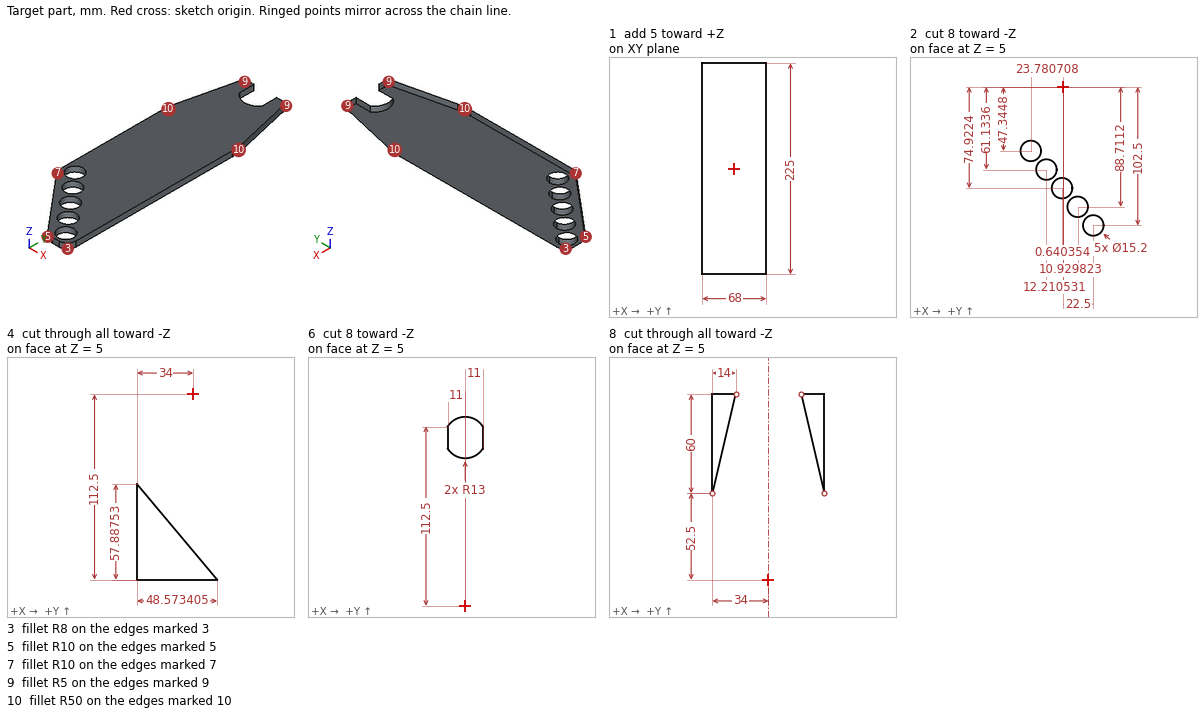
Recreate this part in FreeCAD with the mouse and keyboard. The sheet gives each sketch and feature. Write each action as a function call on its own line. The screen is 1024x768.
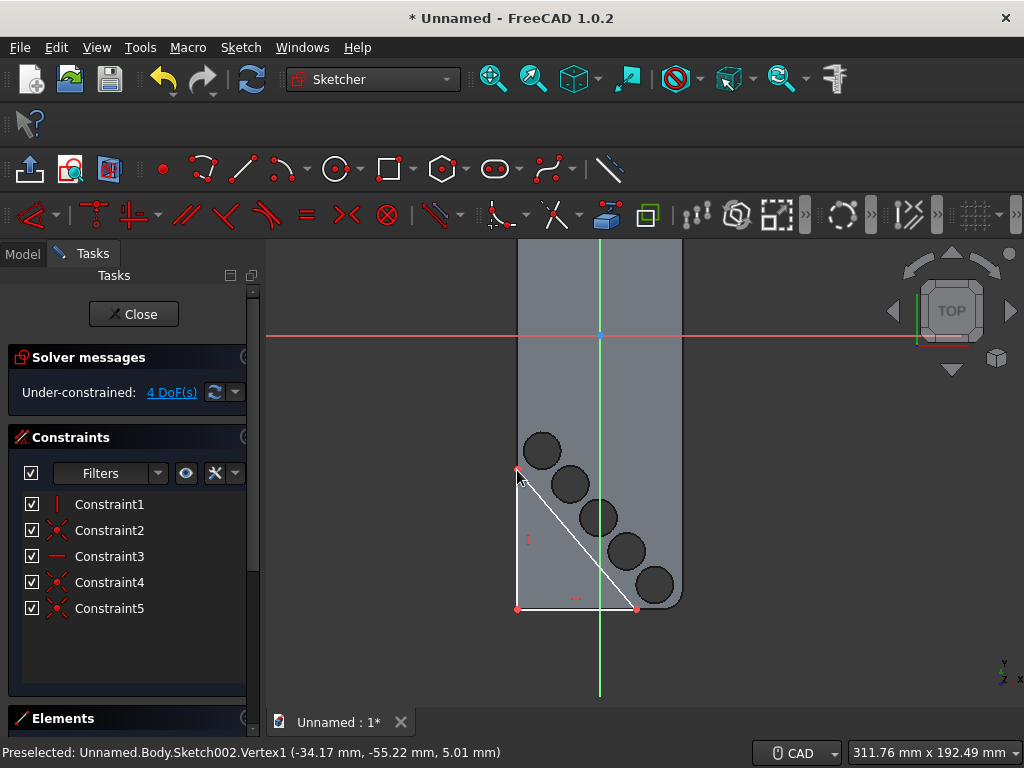
click(32, 216)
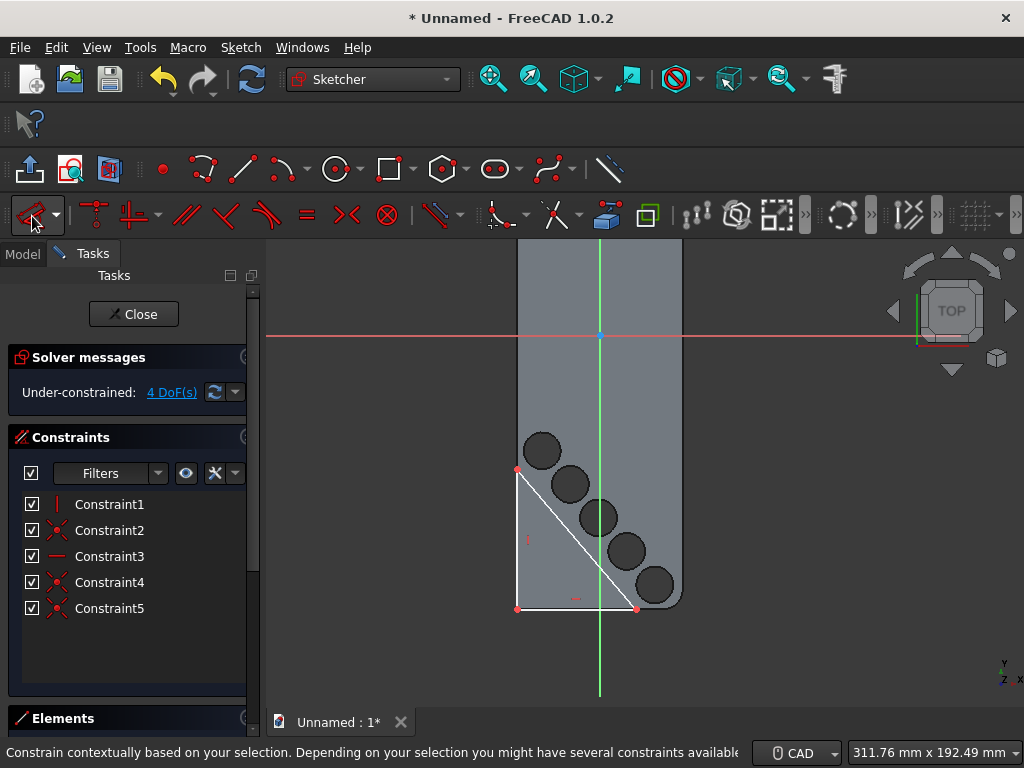
click(517, 470)
click(559, 302)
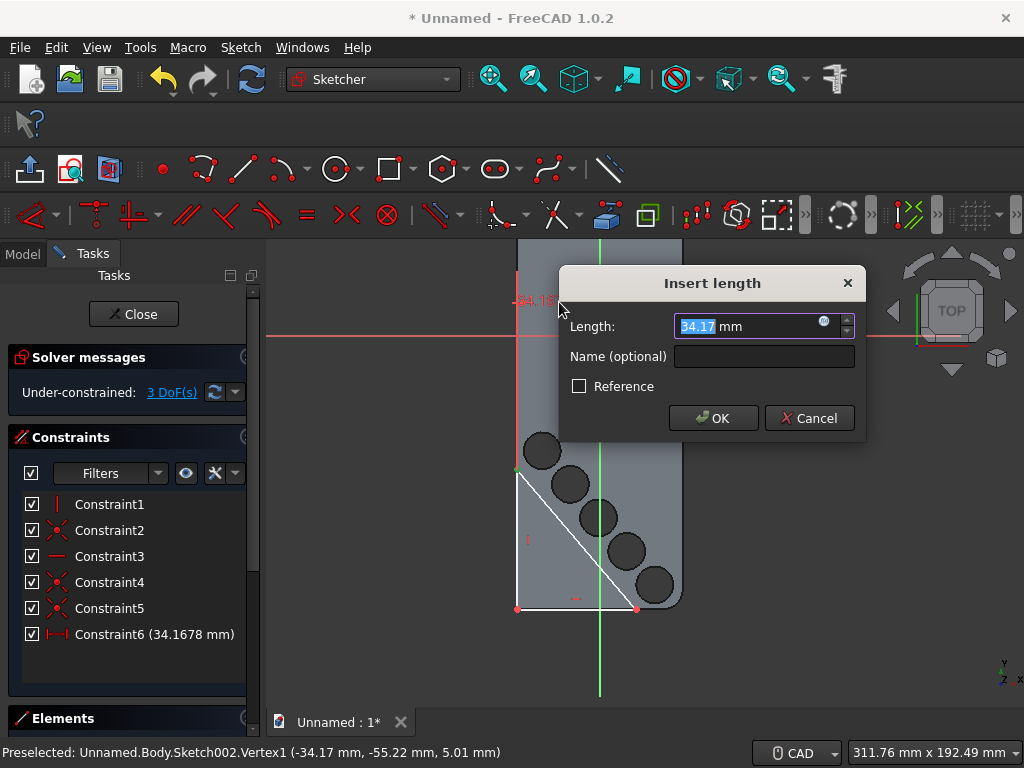
text(34)
key(Return)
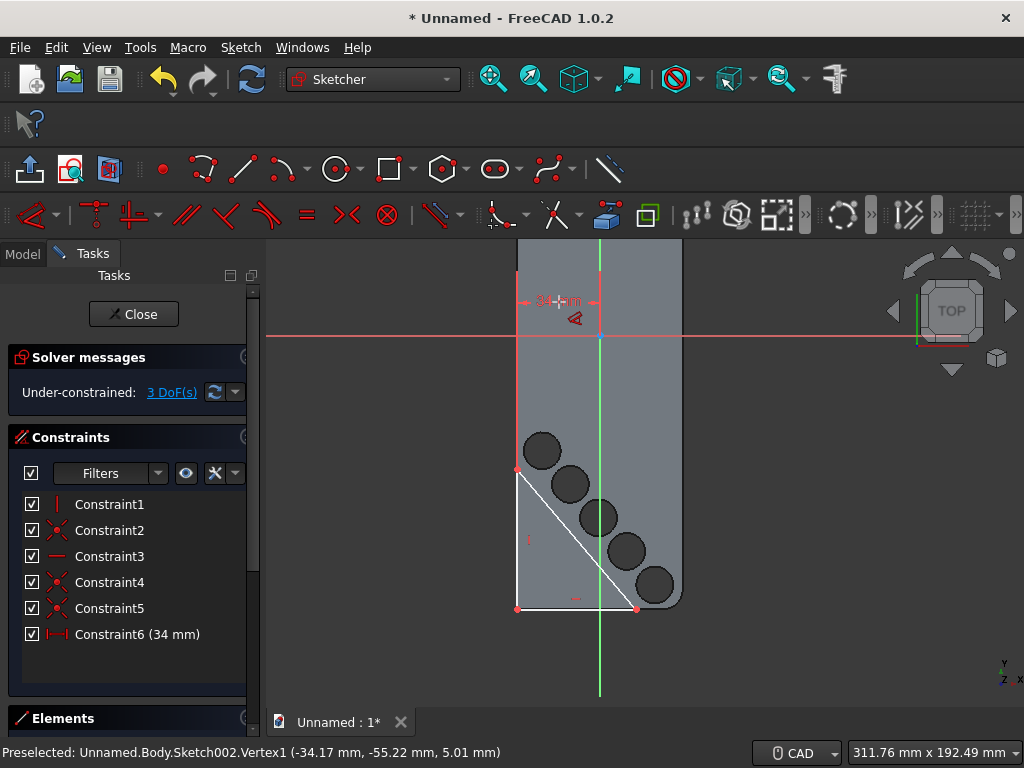
click(517, 610)
click(483, 473)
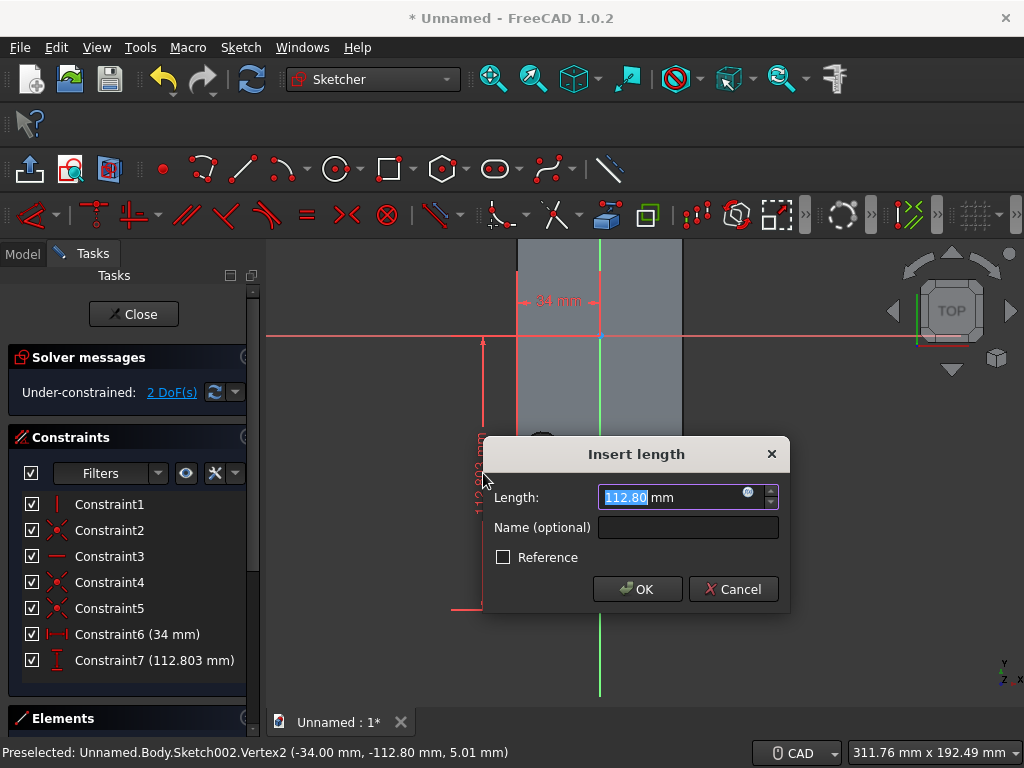
text(112.5)
key(Return)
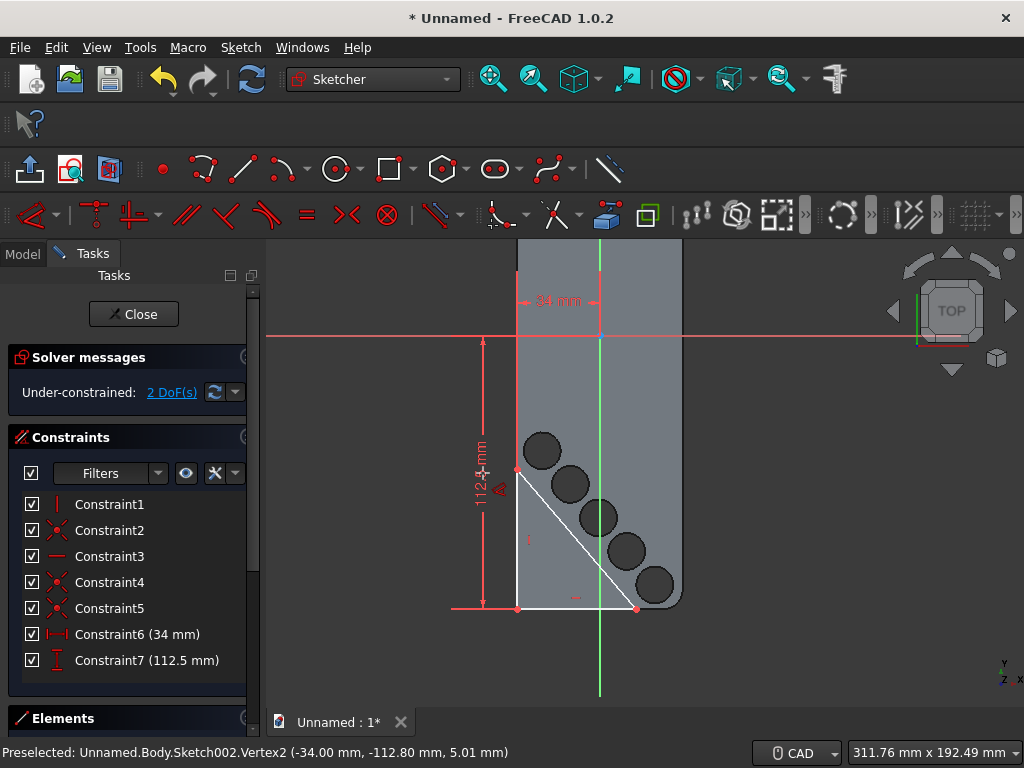
click(517, 512)
click(483, 540)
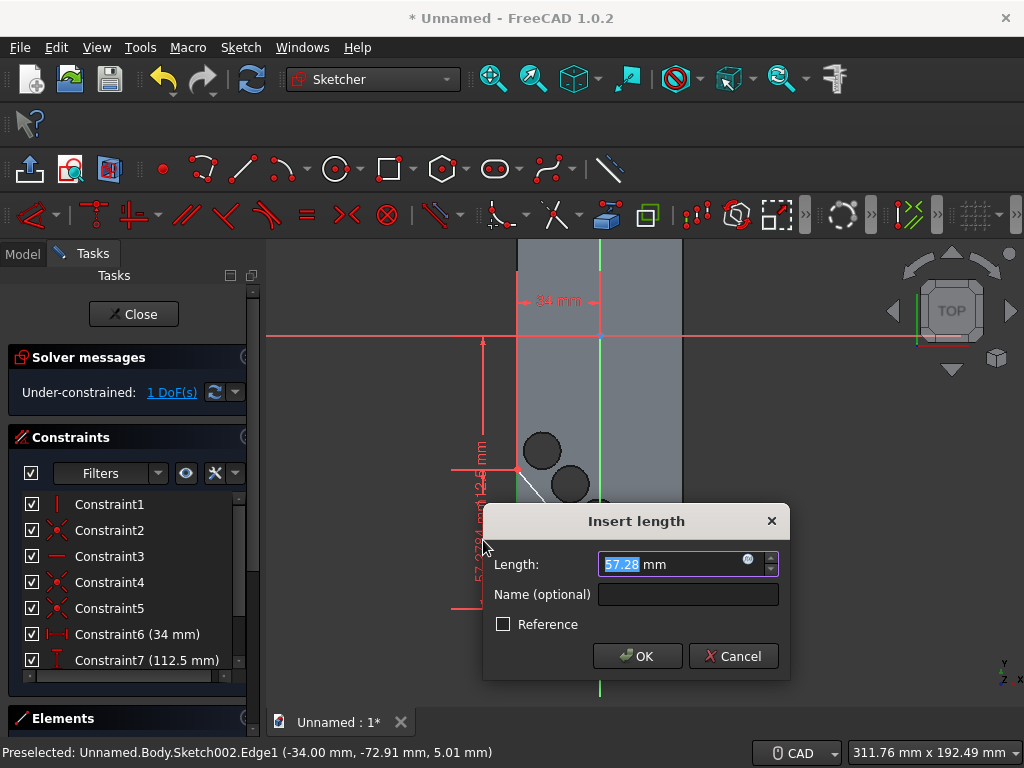
text(57.88753)
key(Return)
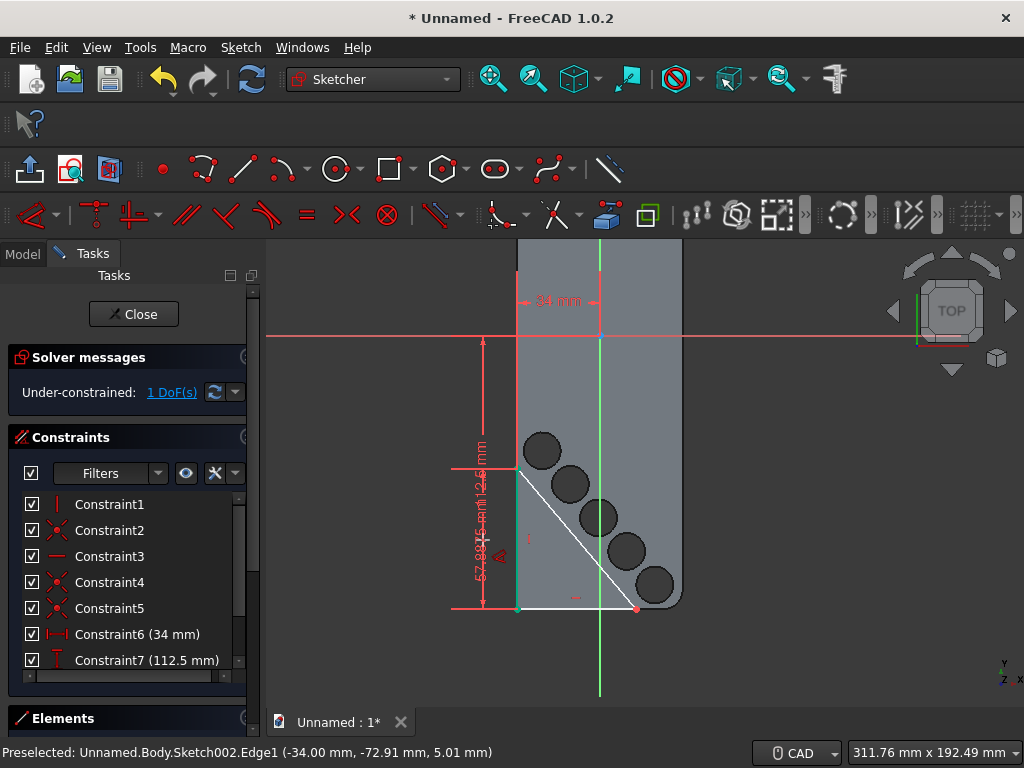
click(553, 609)
click(577, 643)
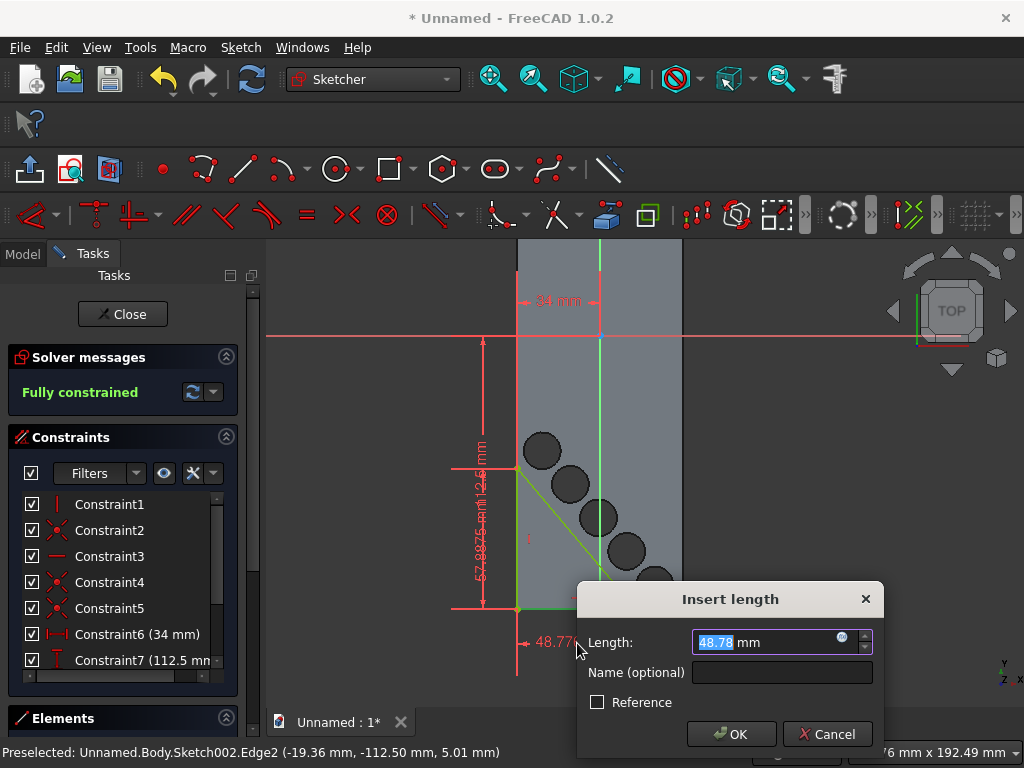
text(48.573405)
key(Return)
key(Escape)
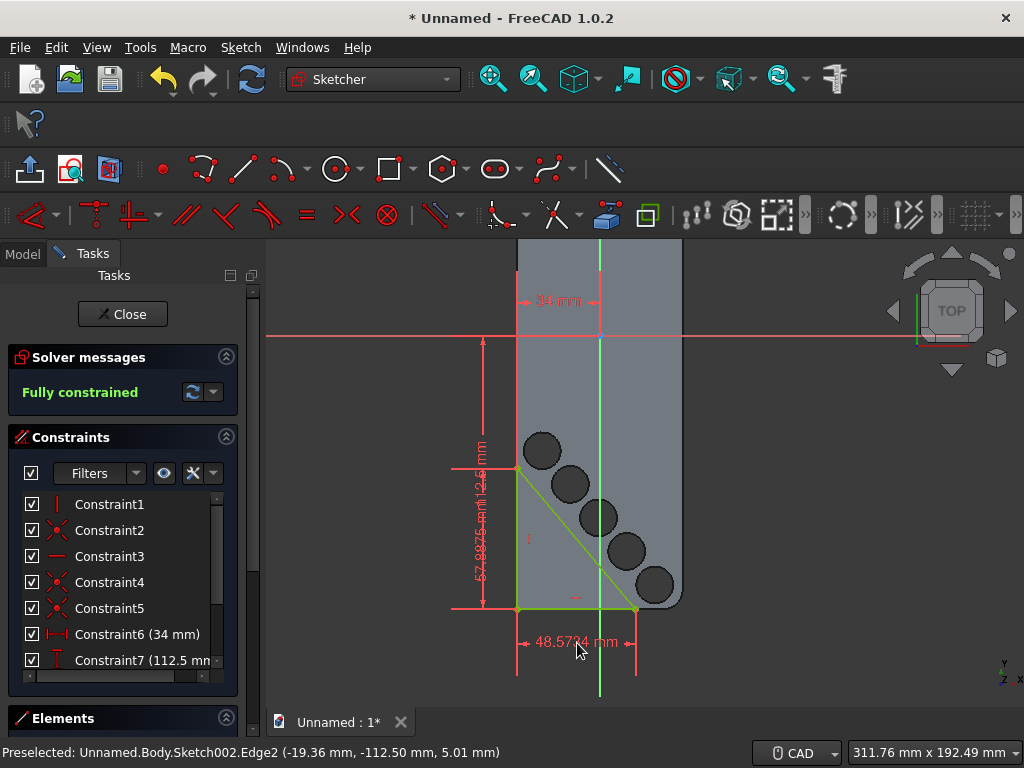
click(123, 314)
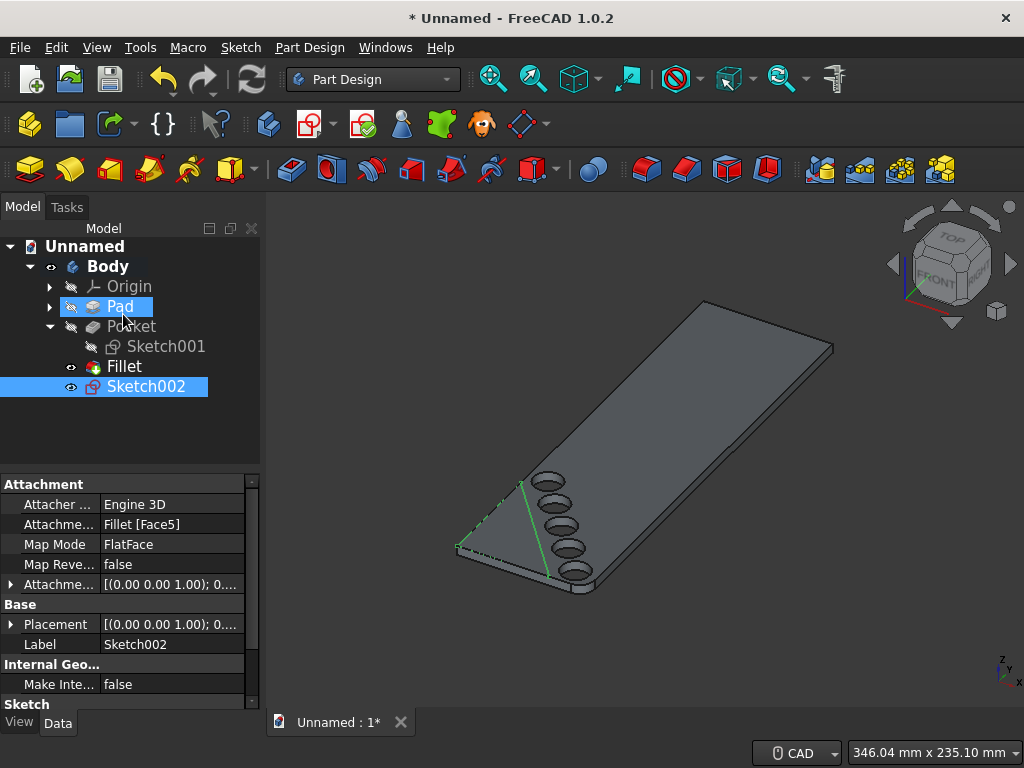
click(292, 170)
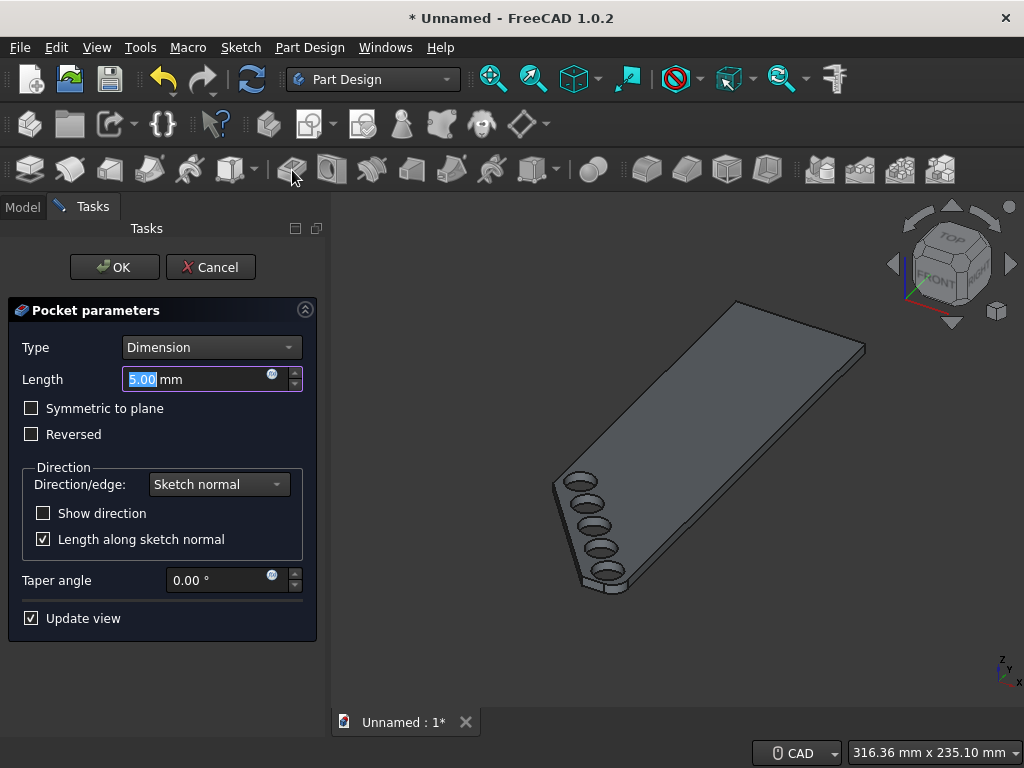
click(212, 348)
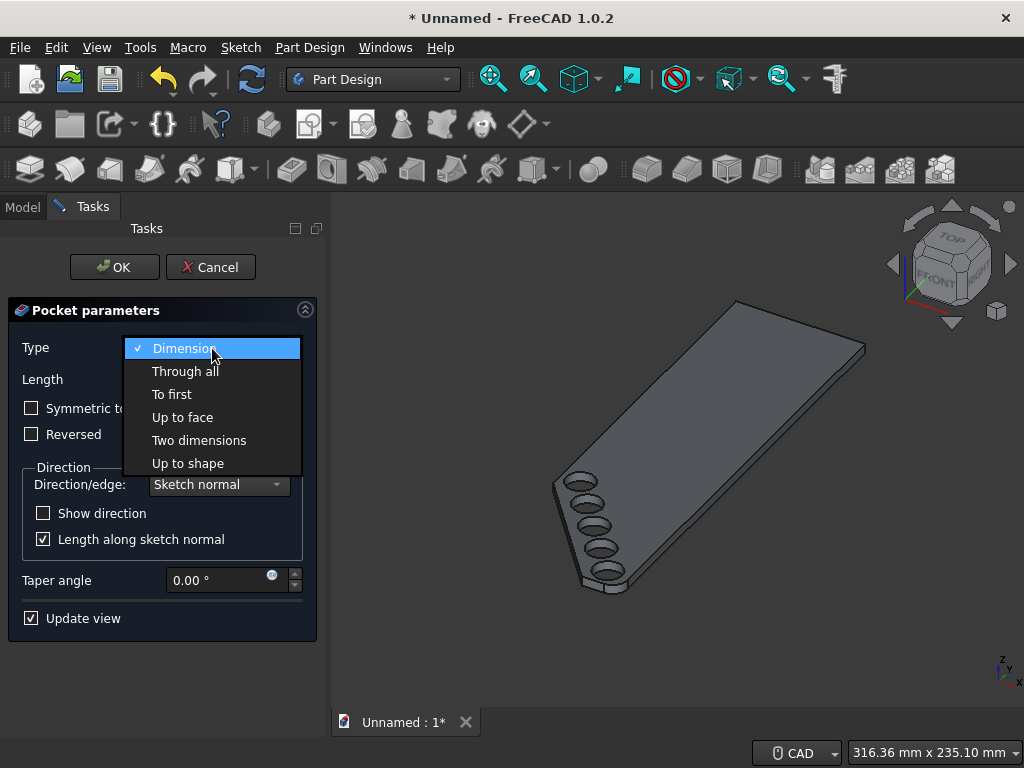
click(212, 372)